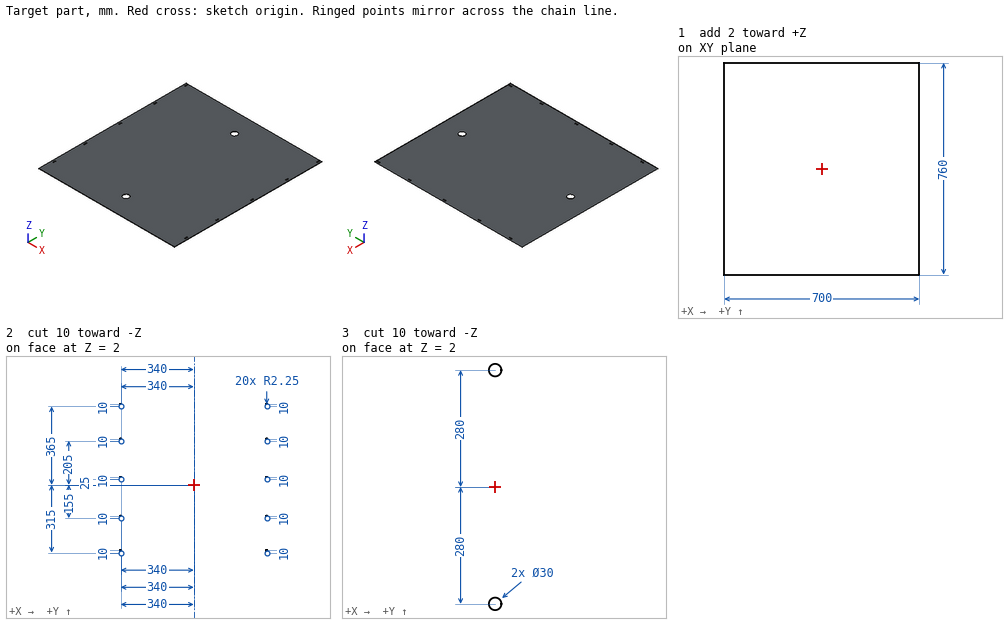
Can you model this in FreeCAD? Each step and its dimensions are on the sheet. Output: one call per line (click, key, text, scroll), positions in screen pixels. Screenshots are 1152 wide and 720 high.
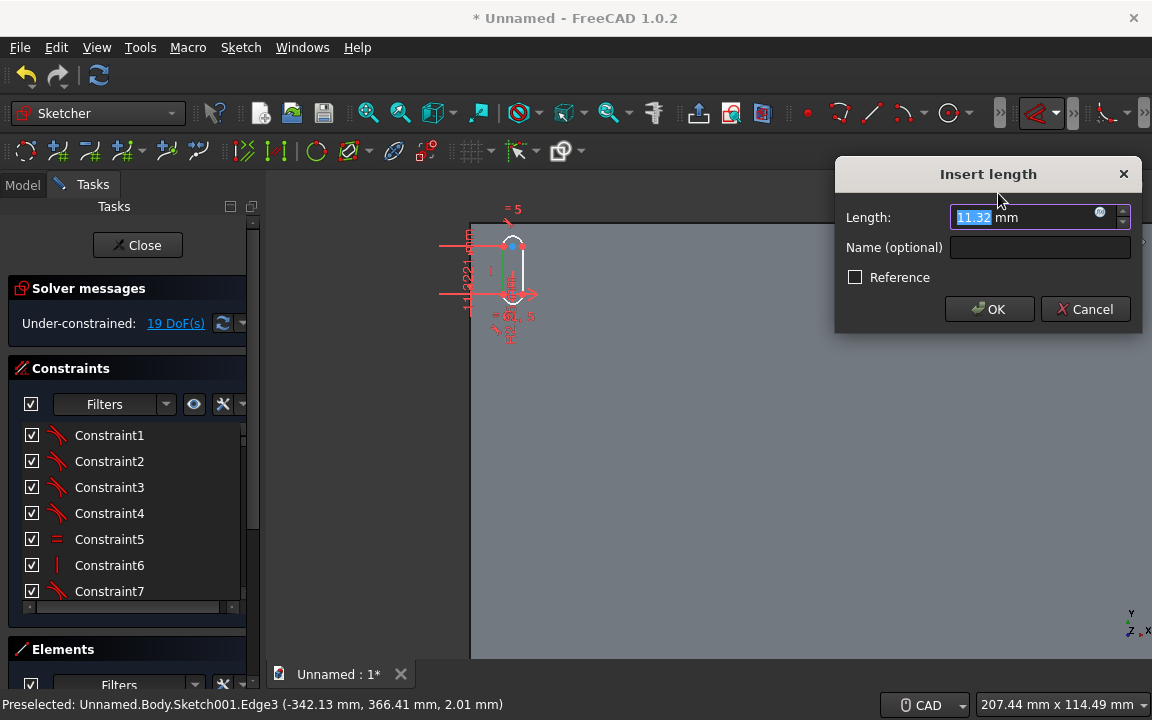
text(10)
key(Return)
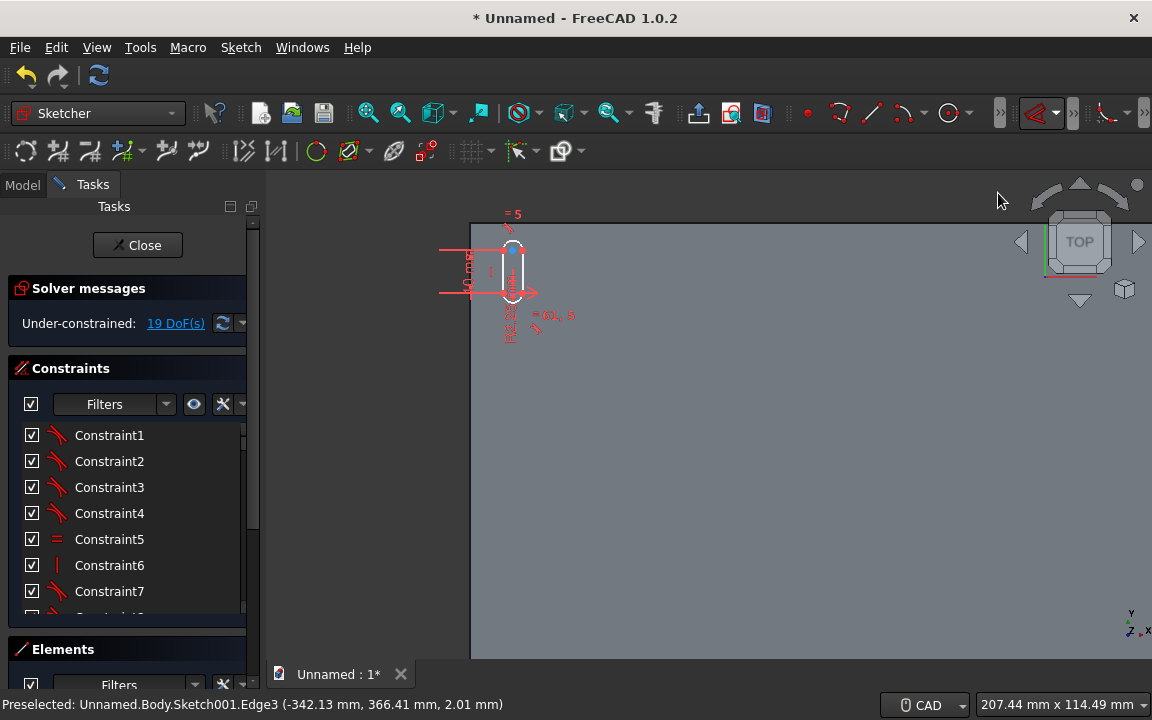
scroll(476, 252, down, 11)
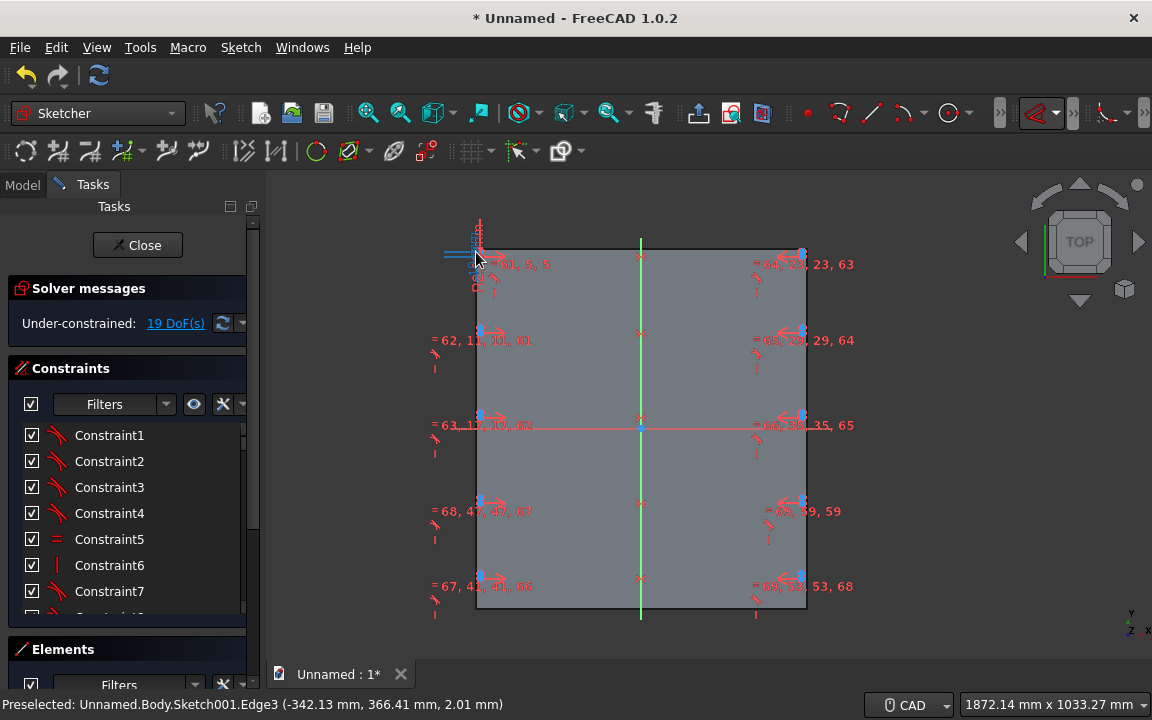
scroll(479, 331, up, 11)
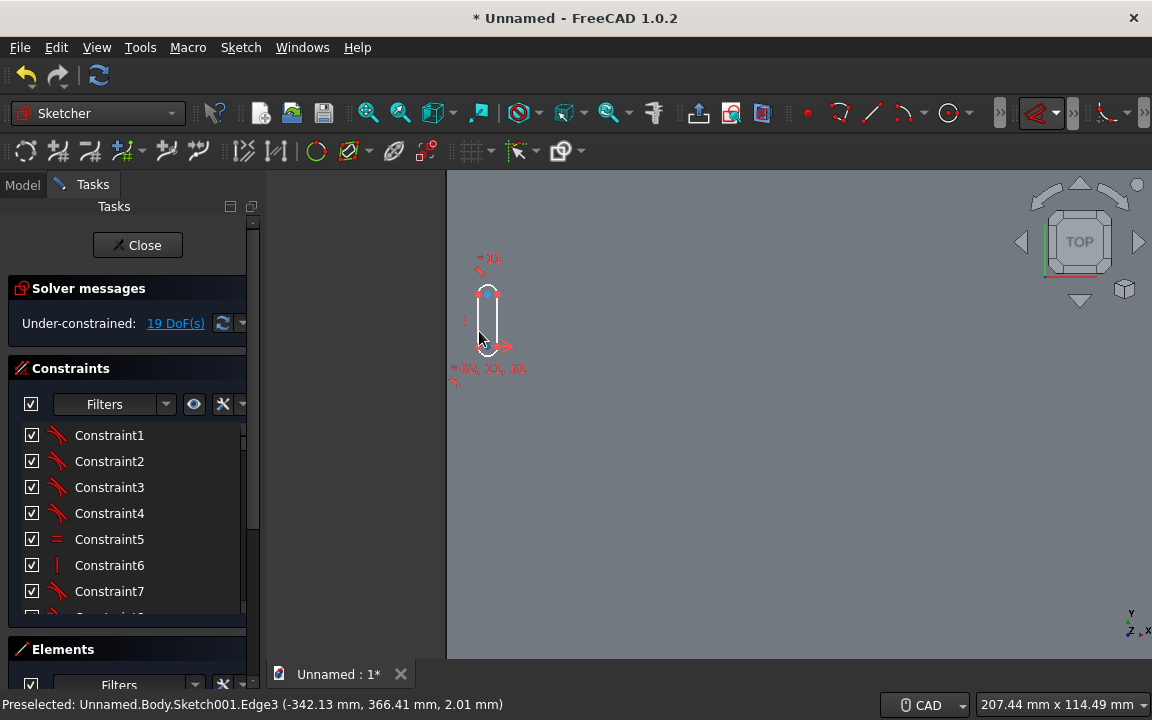
click(478, 331)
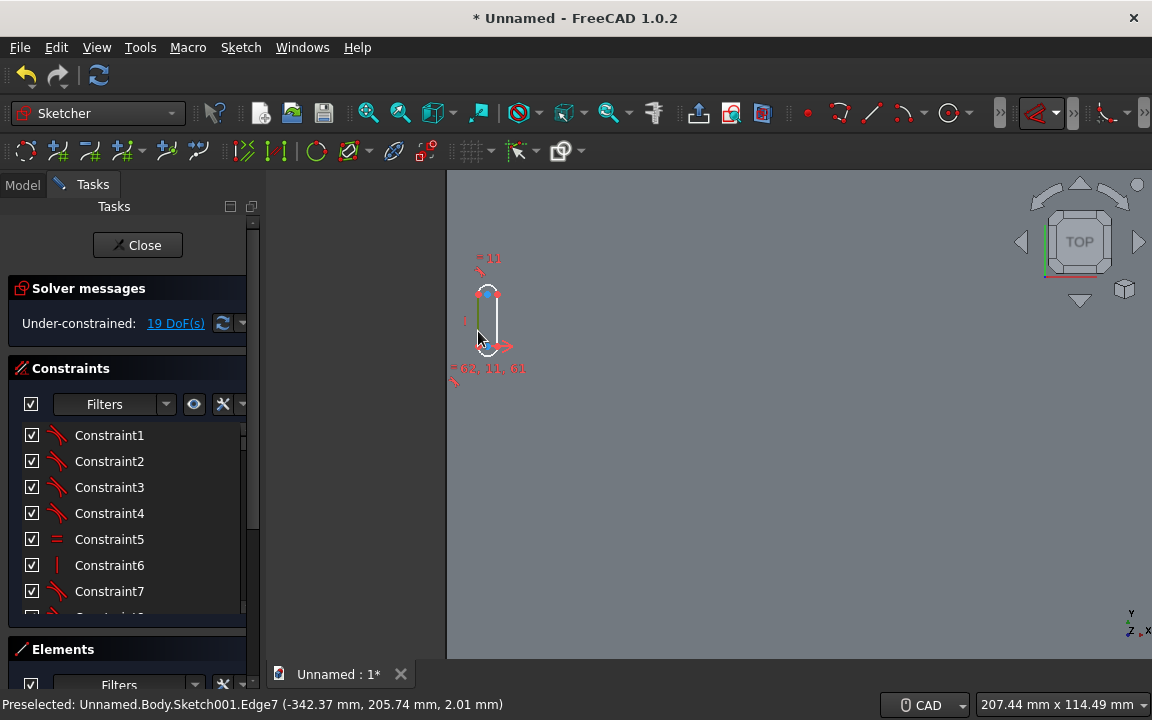
click(1058, 114)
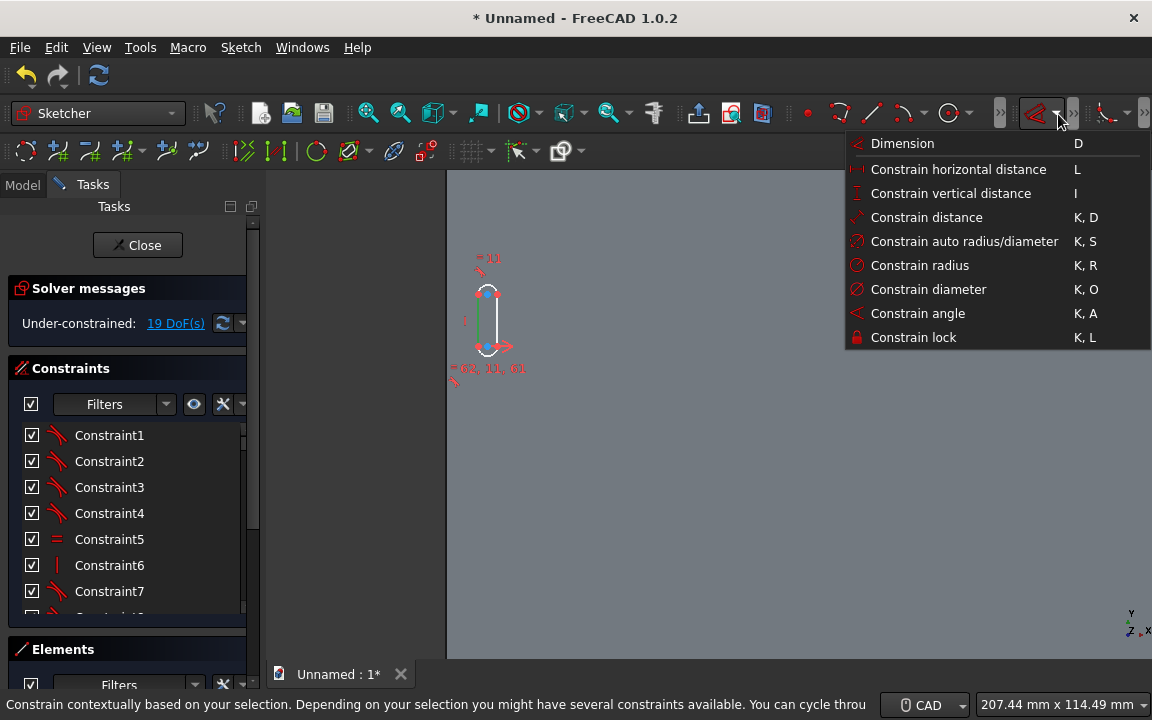
click(998, 193)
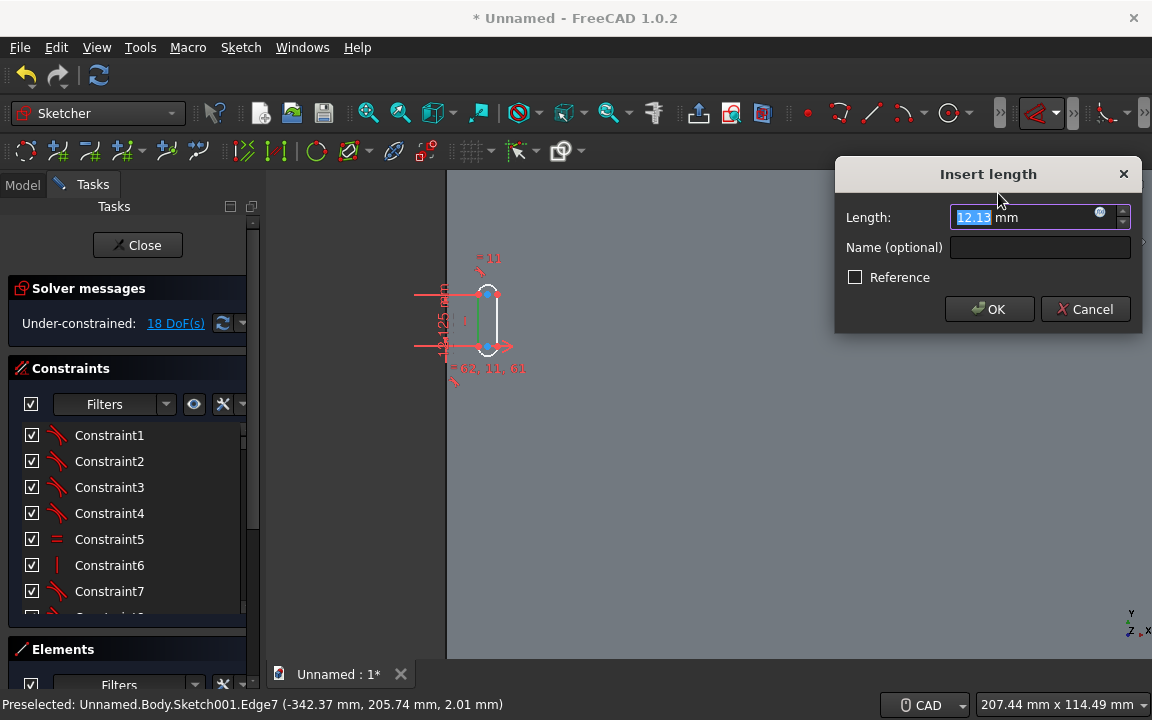
text(10)
key(Return)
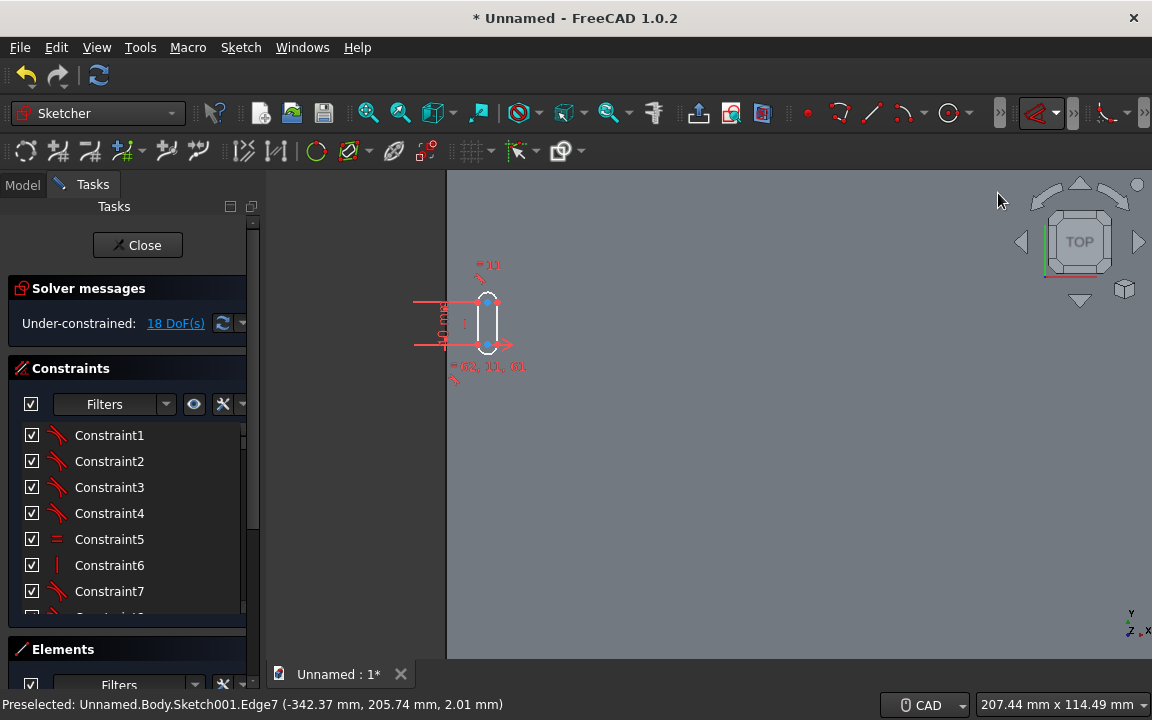
scroll(479, 331, down, 11)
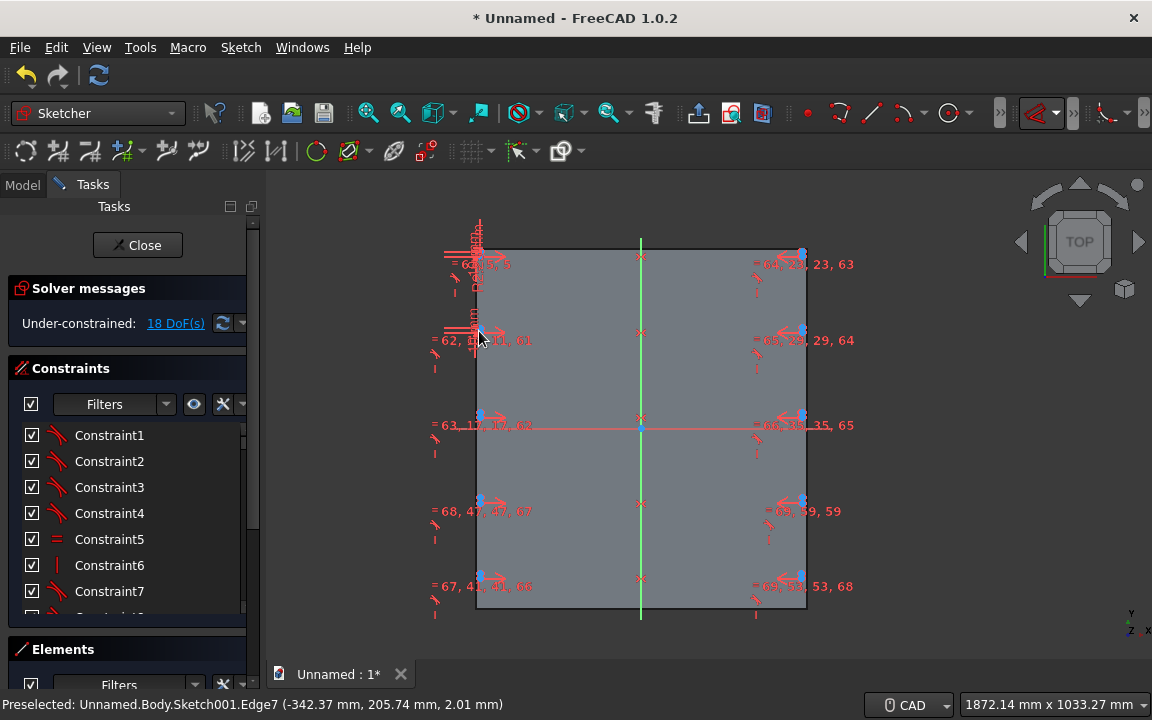
scroll(479, 416, up, 11)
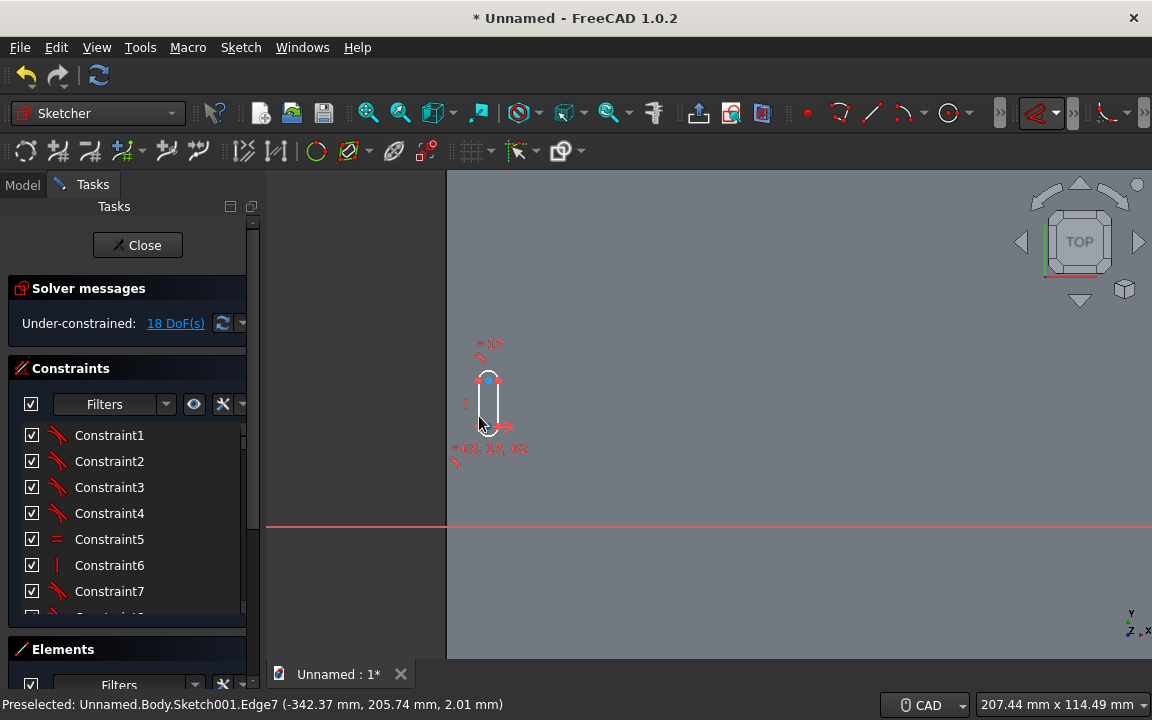
click(479, 413)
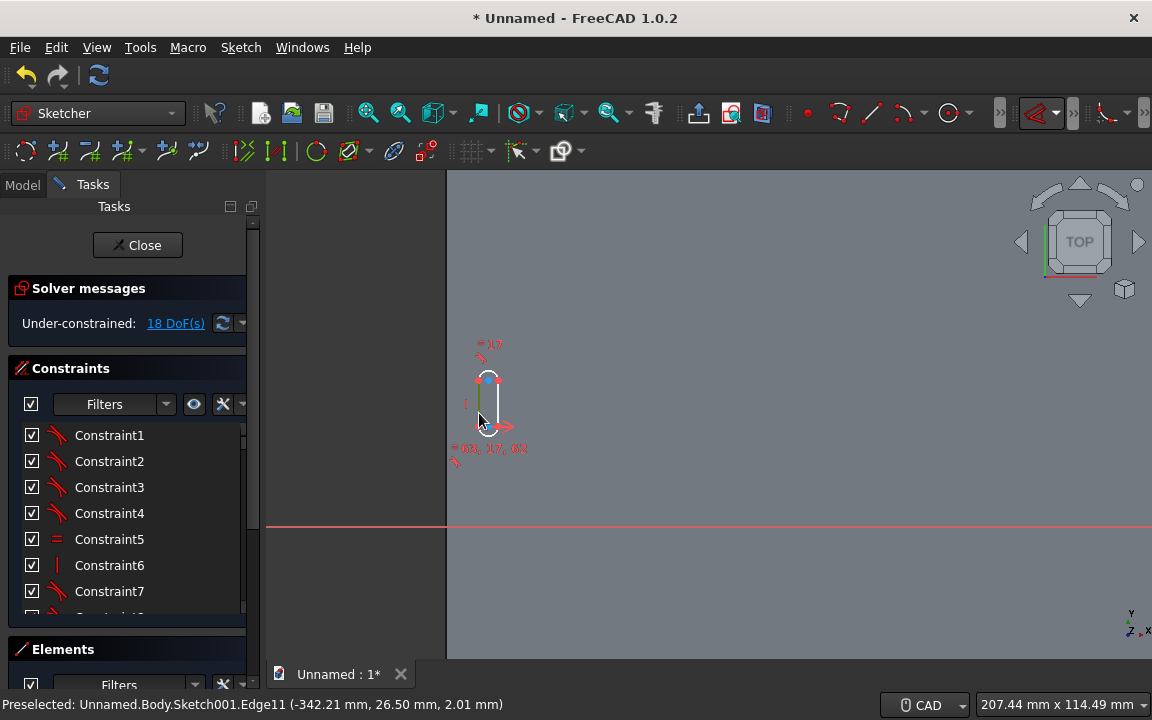
click(1058, 114)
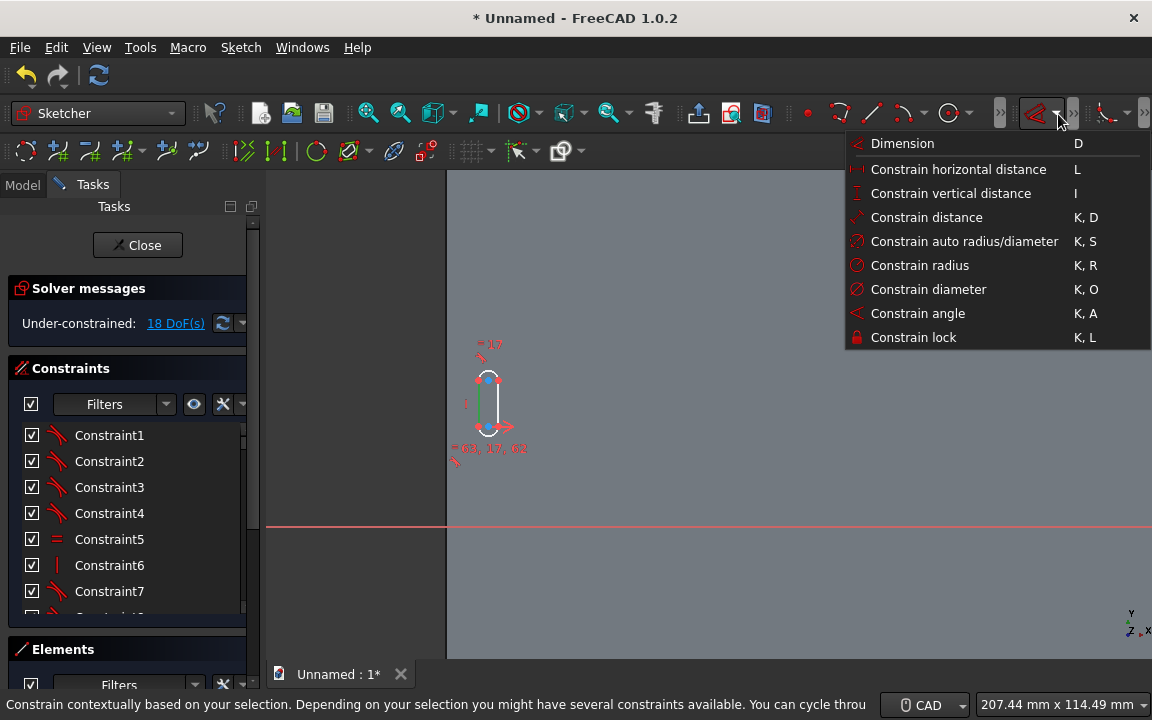
click(998, 193)